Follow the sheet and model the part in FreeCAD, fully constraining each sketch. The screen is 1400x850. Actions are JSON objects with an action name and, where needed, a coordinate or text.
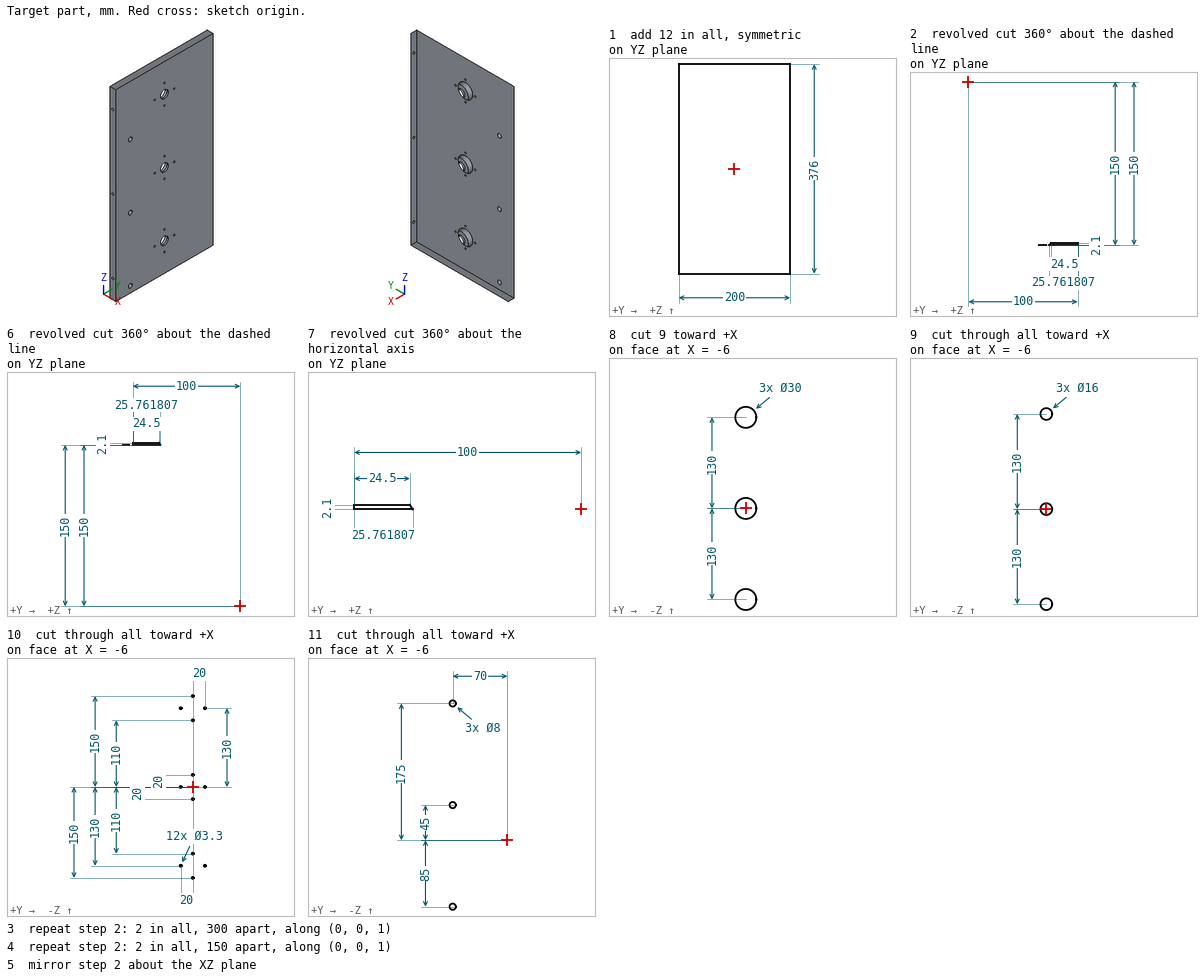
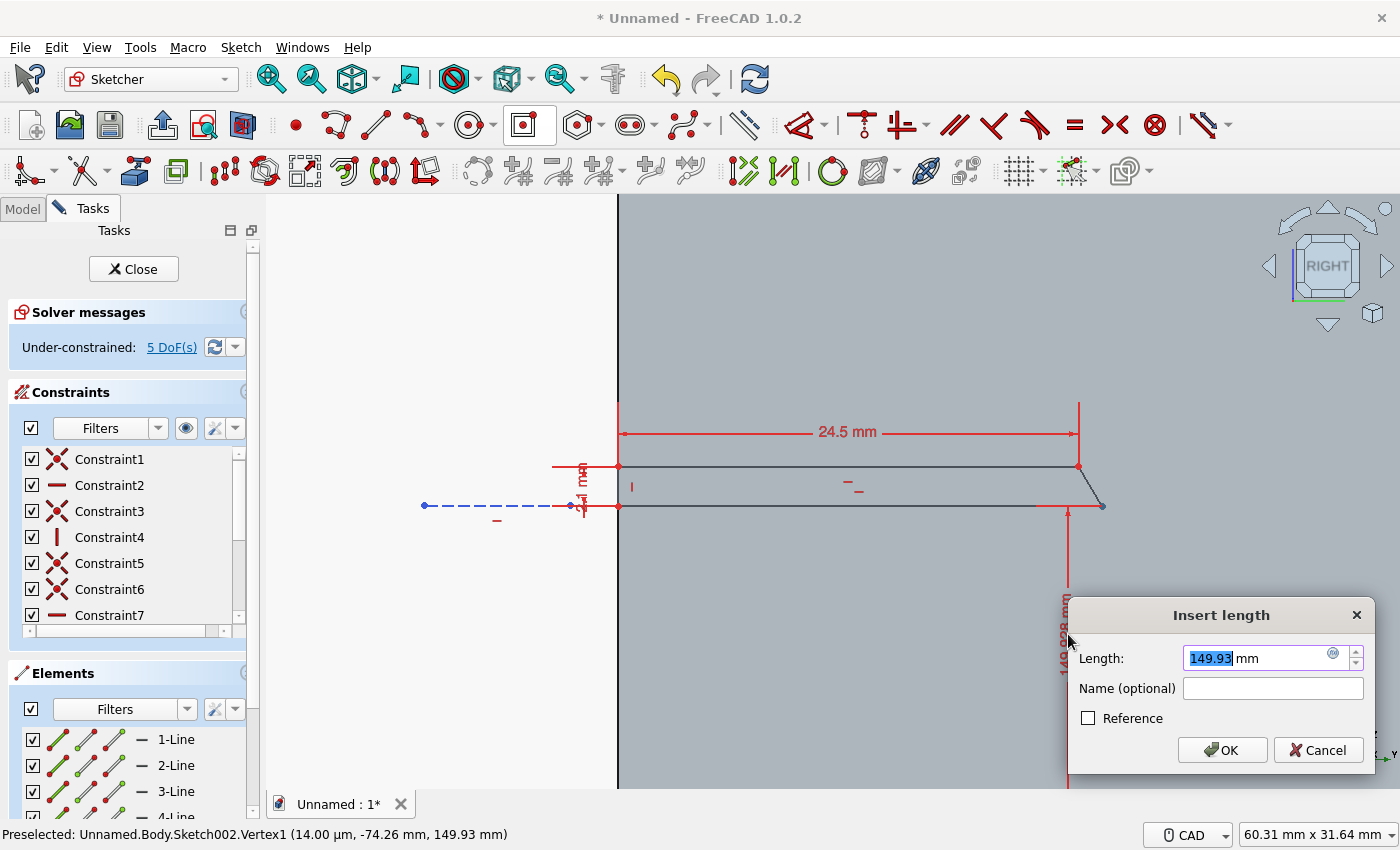
{"action": "type", "text": "150"}
{"action": "key", "text": "Return"}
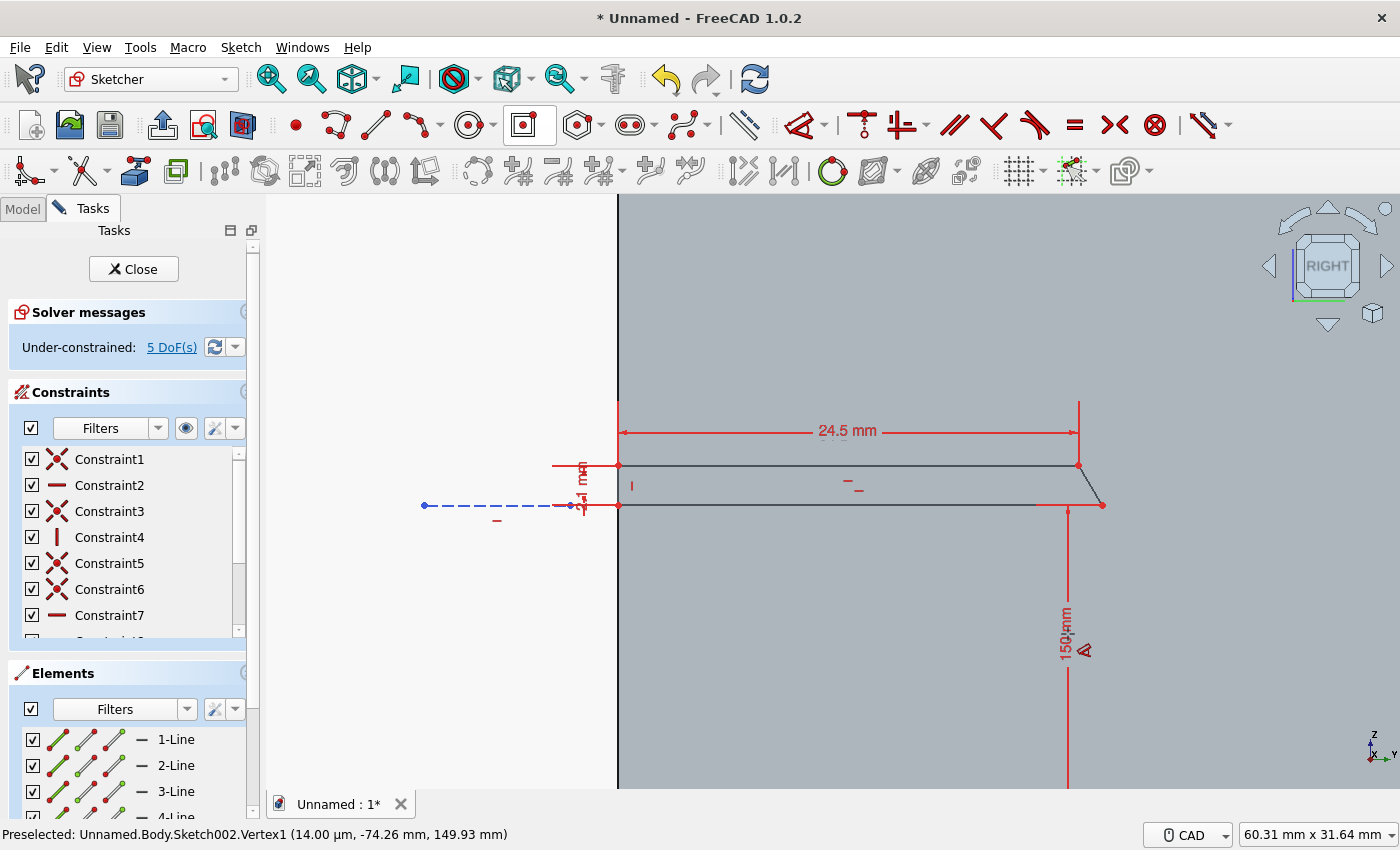
{"action": "left_click", "coordinate": [618, 466]}
{"action": "left_click", "coordinate": [926, 432]}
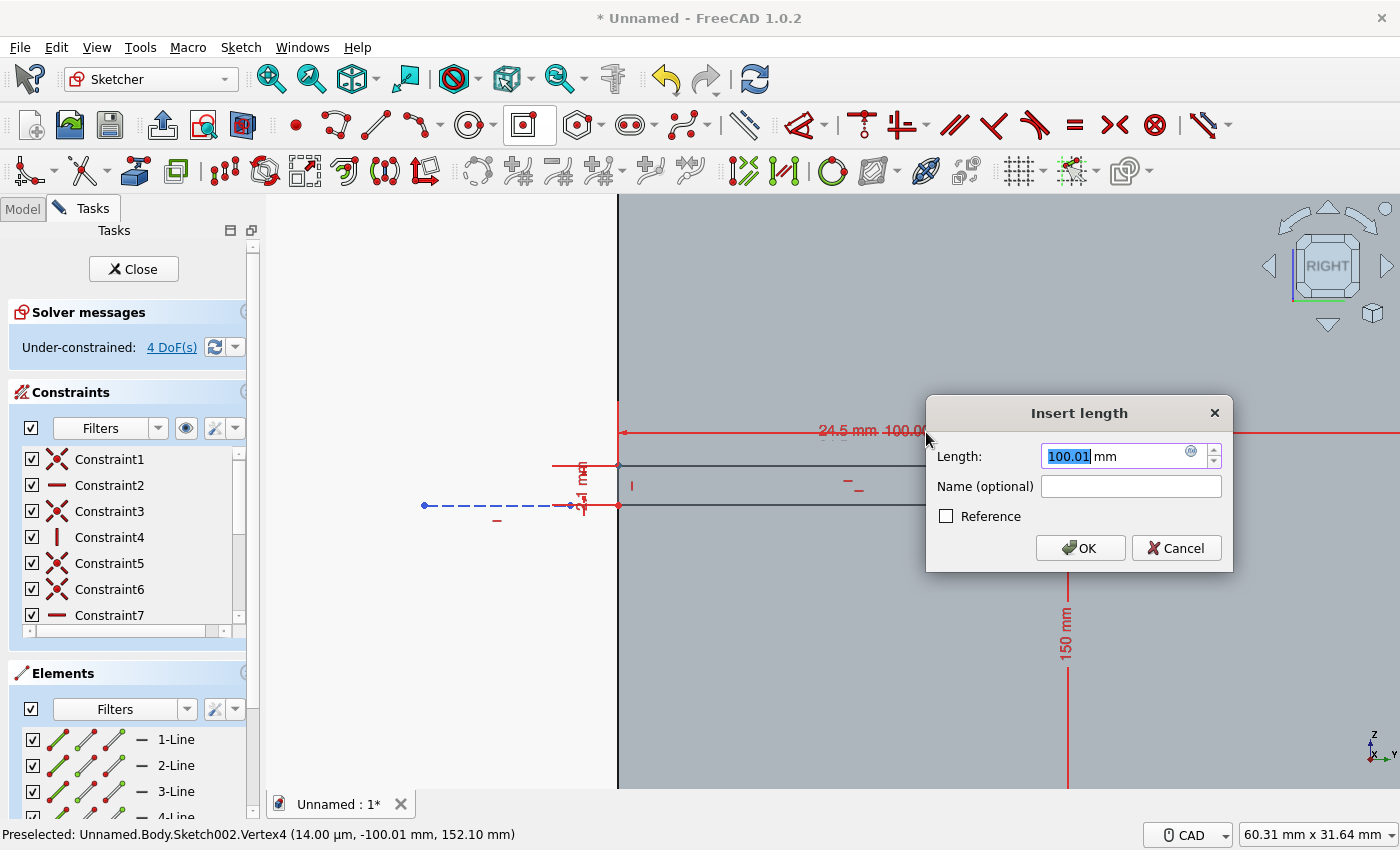
{"action": "type", "text": "100"}
{"action": "key", "text": "Return"}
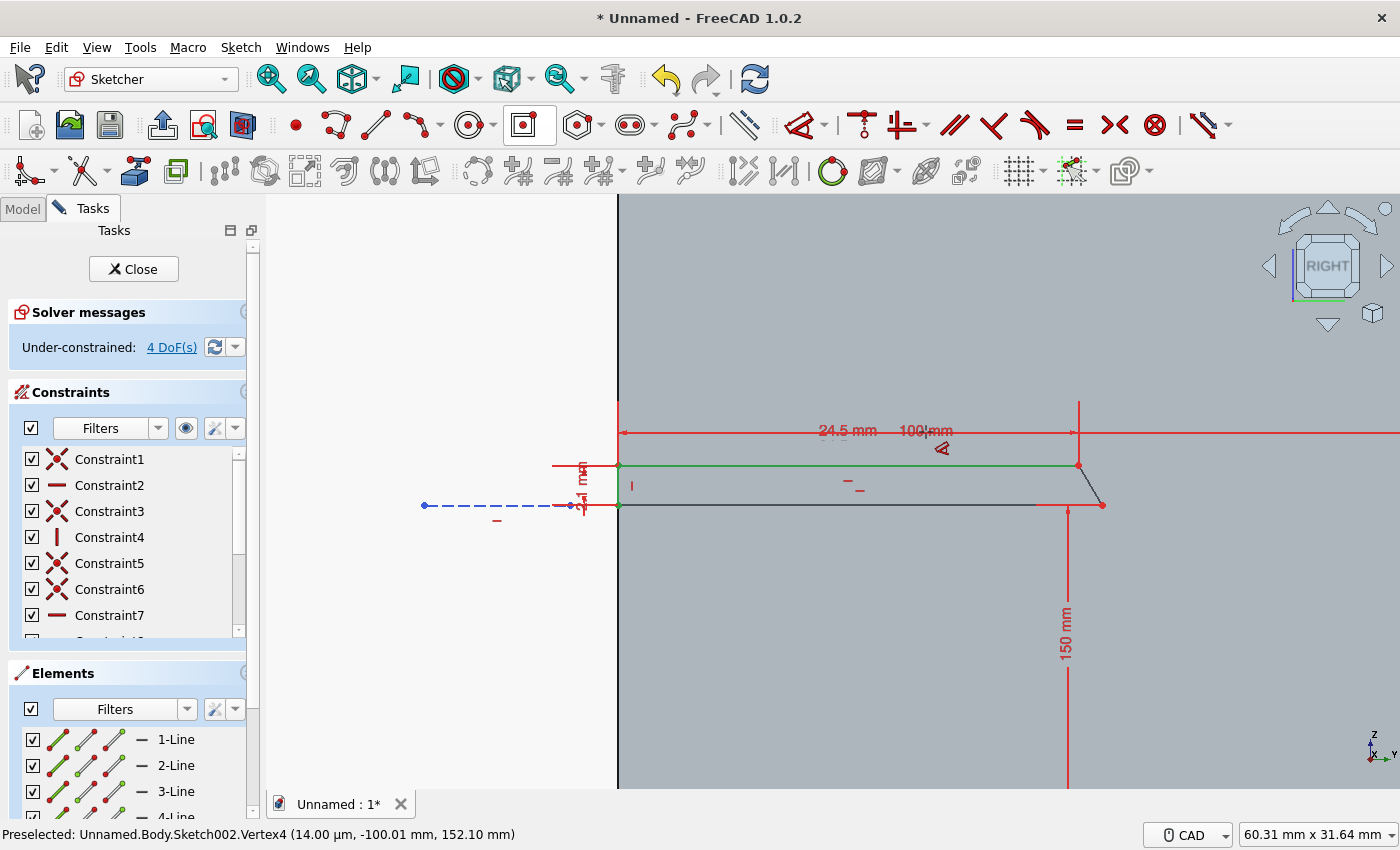
{"action": "left_click", "coordinate": [570, 506]}
{"action": "left_click", "coordinate": [536, 633]}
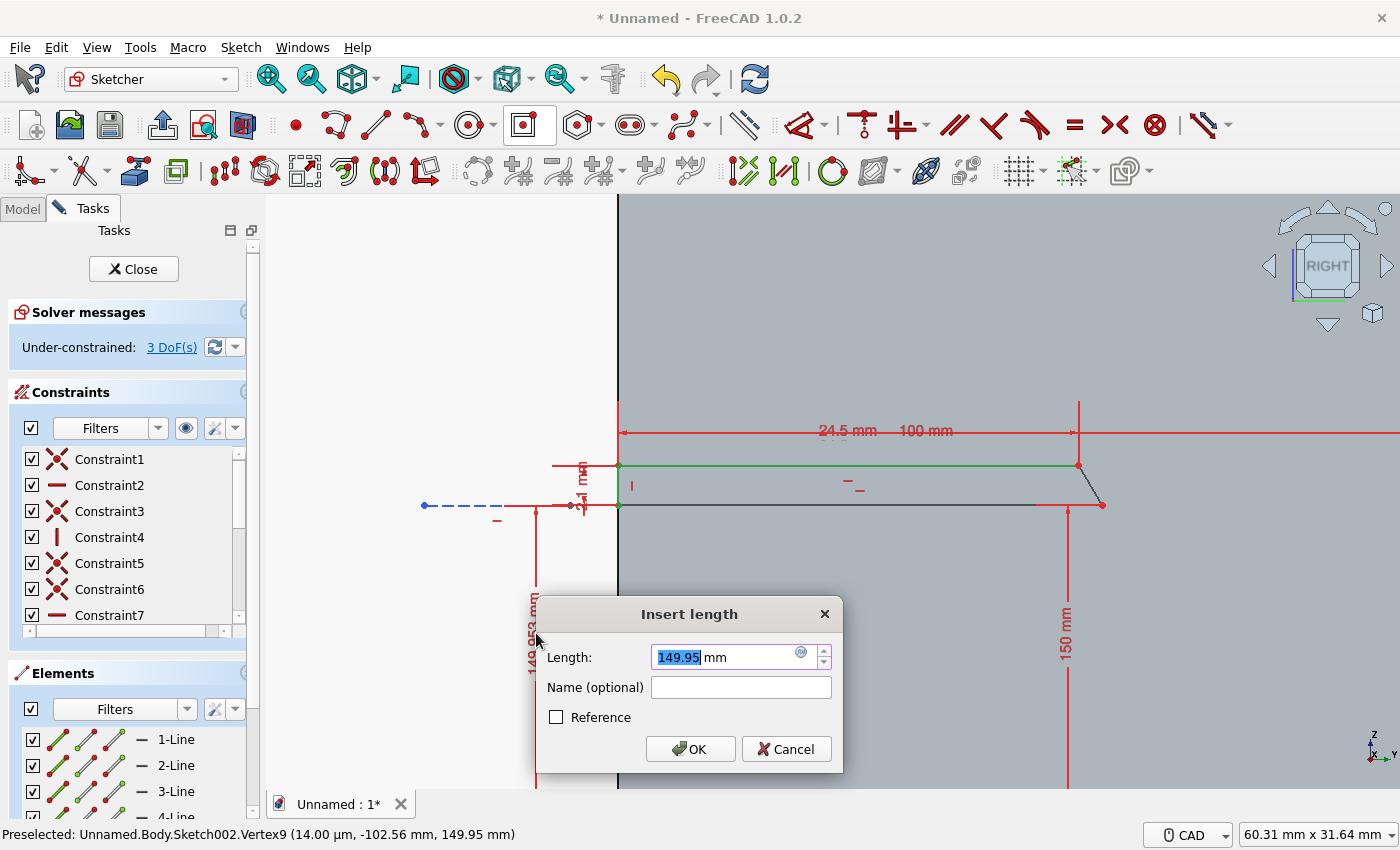
{"action": "type", "text": "150"}
{"action": "key", "text": "Return"}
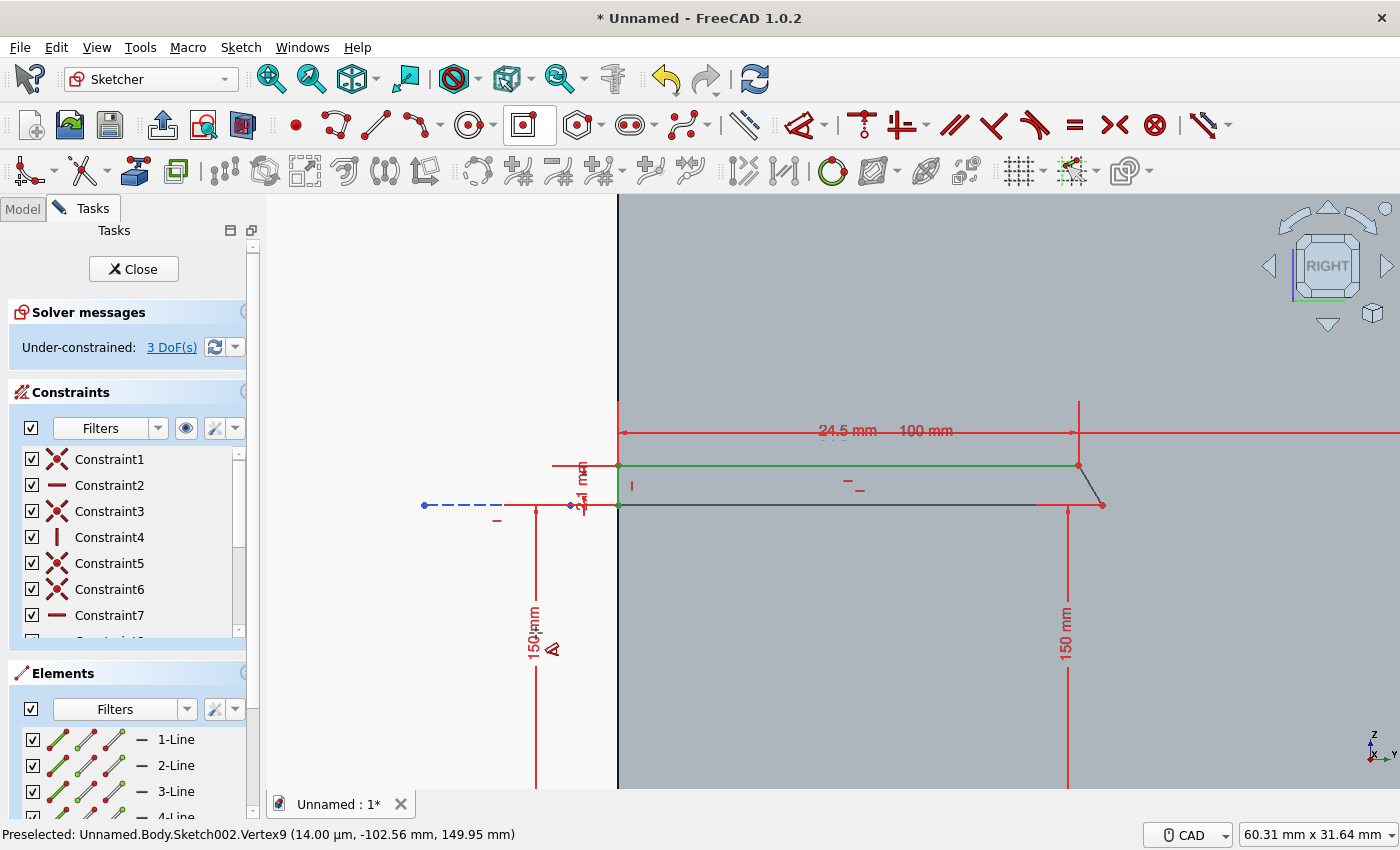
{"action": "left_click", "coordinate": [763, 505]}
{"action": "left_click", "coordinate": [860, 539]}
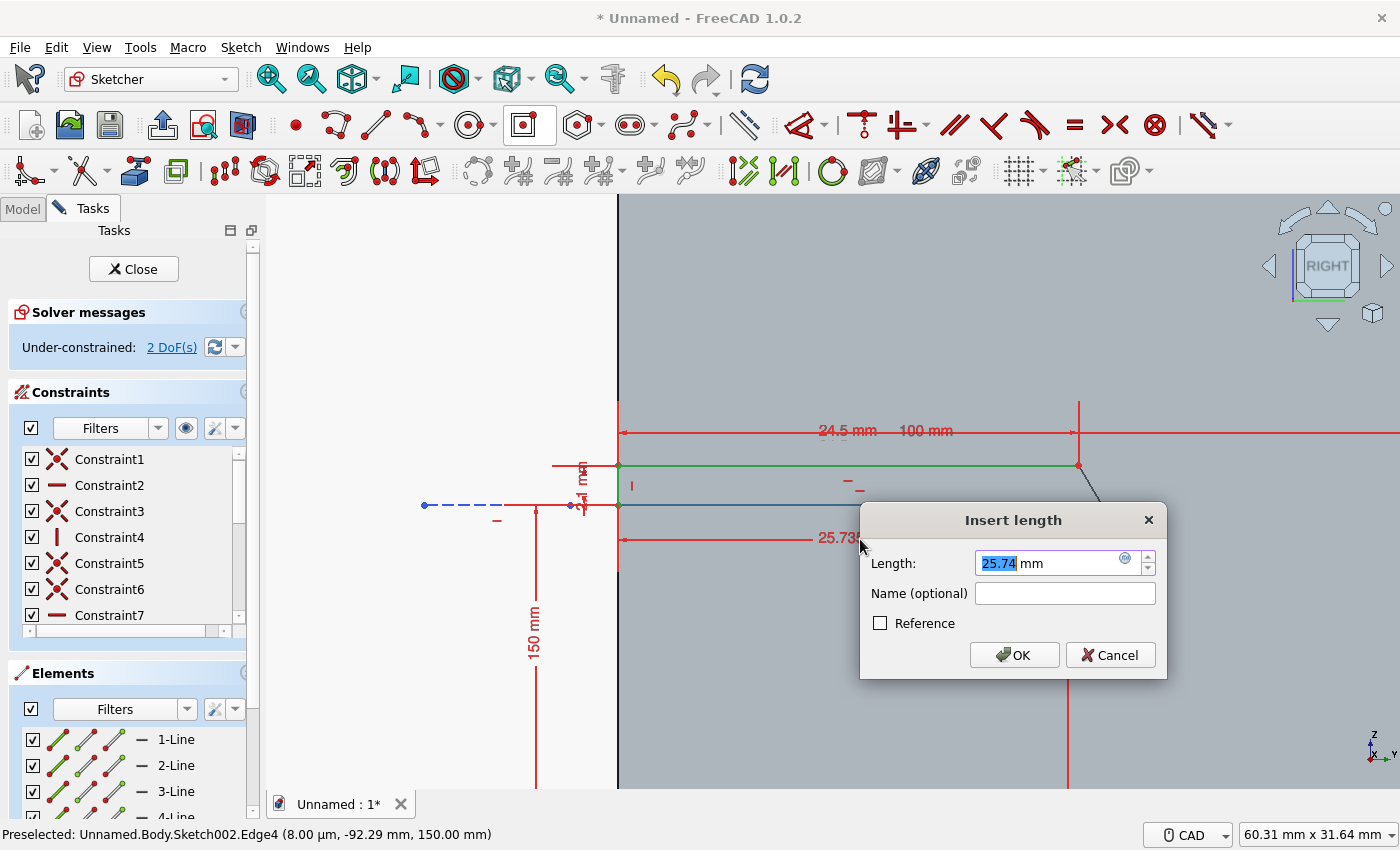
{"action": "type", "text": "25.761807"}
{"action": "key", "text": "Return"}
{"action": "key", "text": "Escape"}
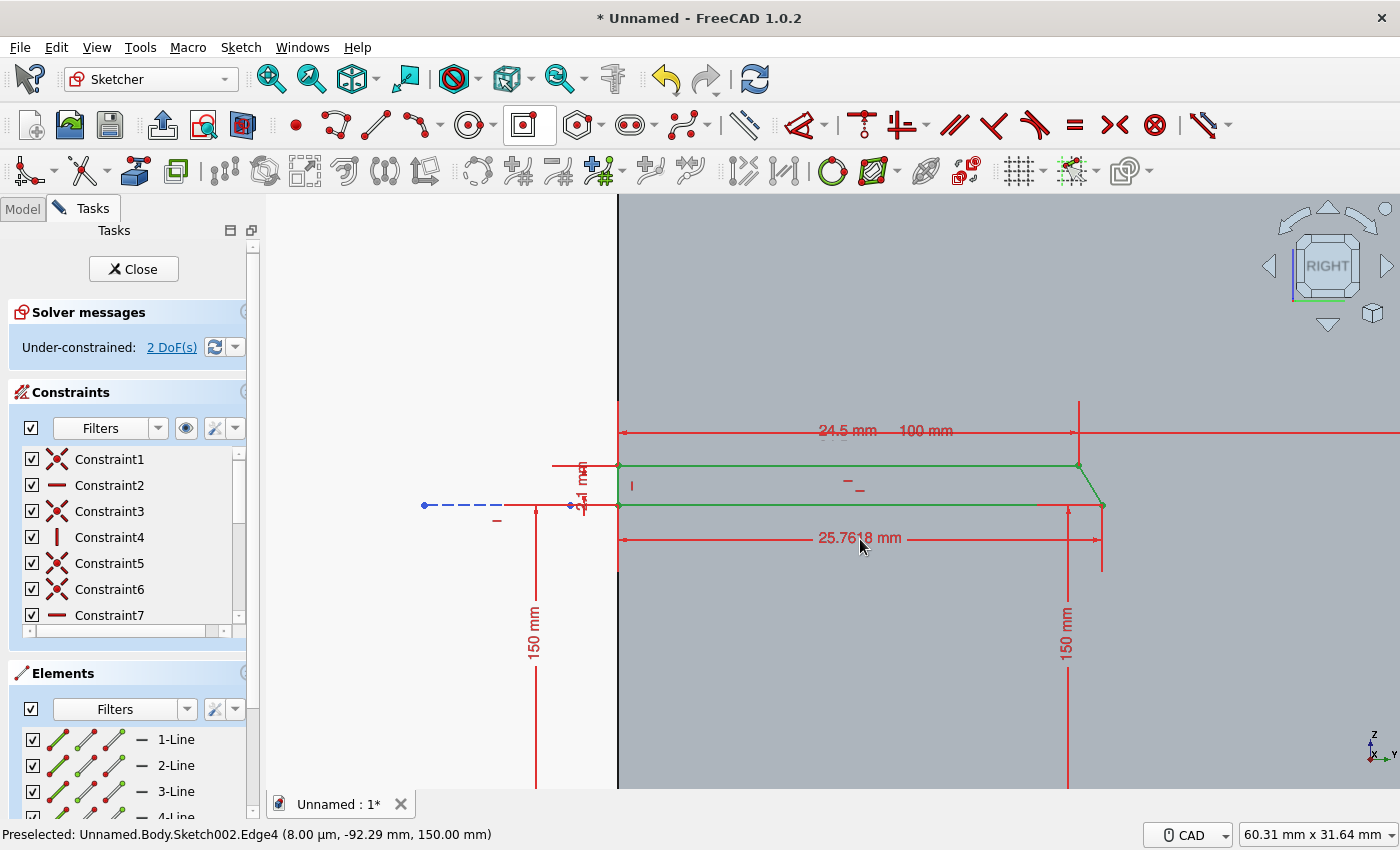
{"action": "left_click", "coordinate": [134, 269]}